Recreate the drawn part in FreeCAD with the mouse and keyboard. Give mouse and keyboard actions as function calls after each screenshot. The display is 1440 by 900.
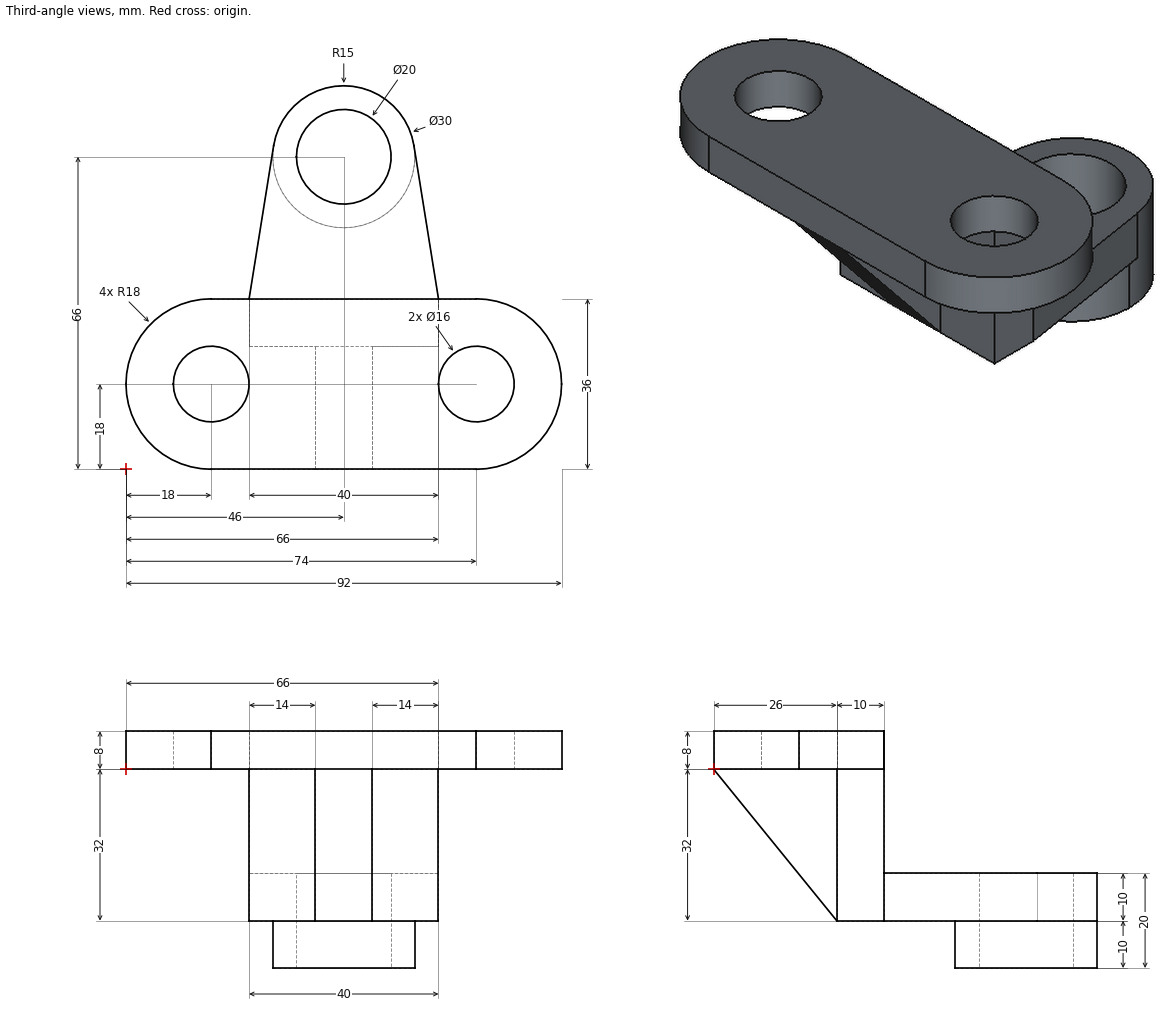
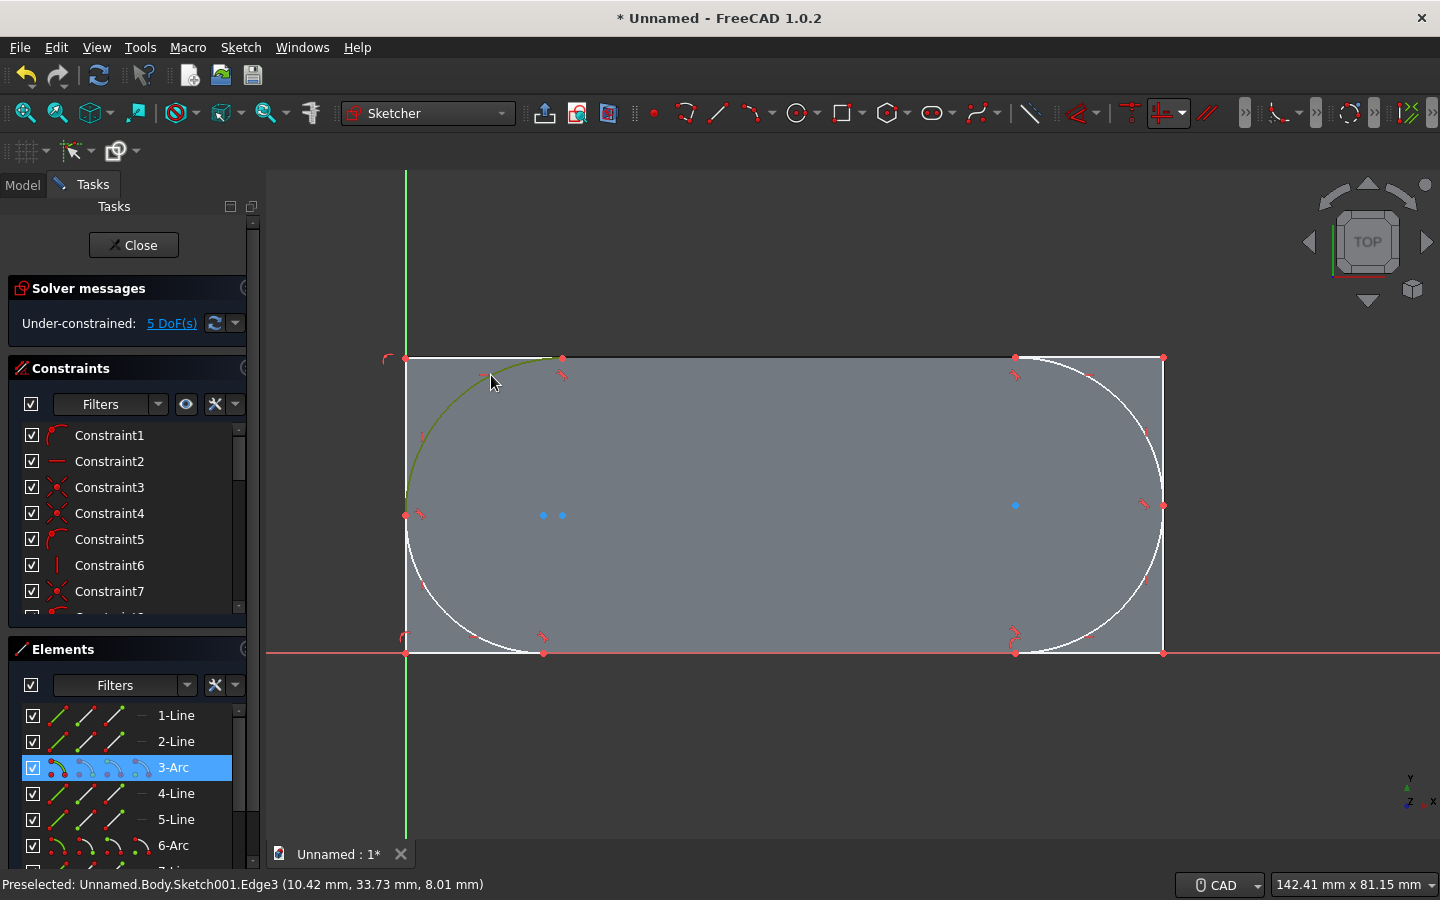
click(481, 638)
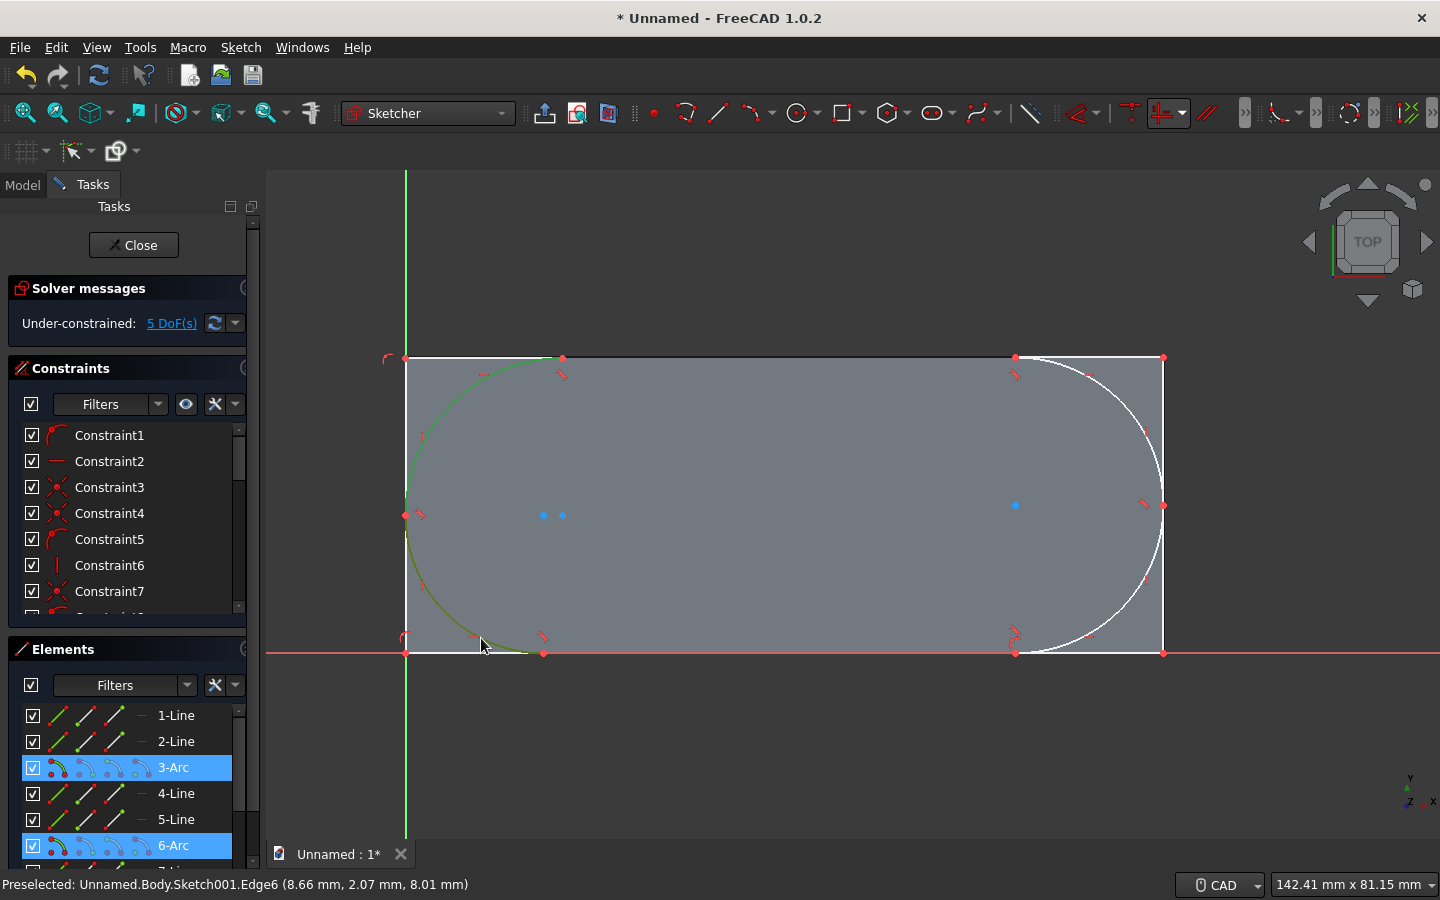
click(1083, 637)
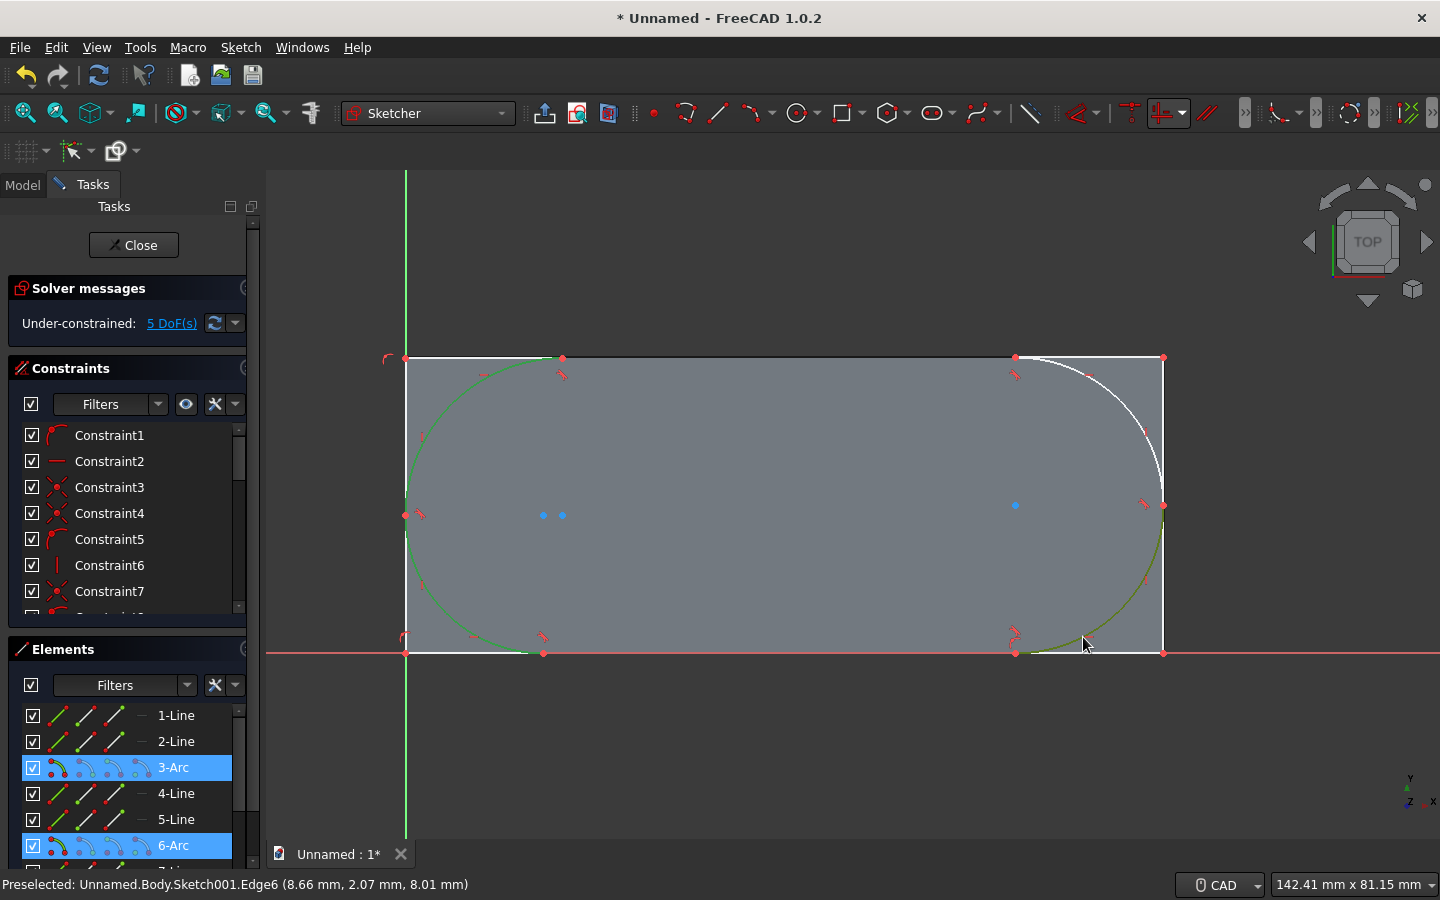
click(1147, 438)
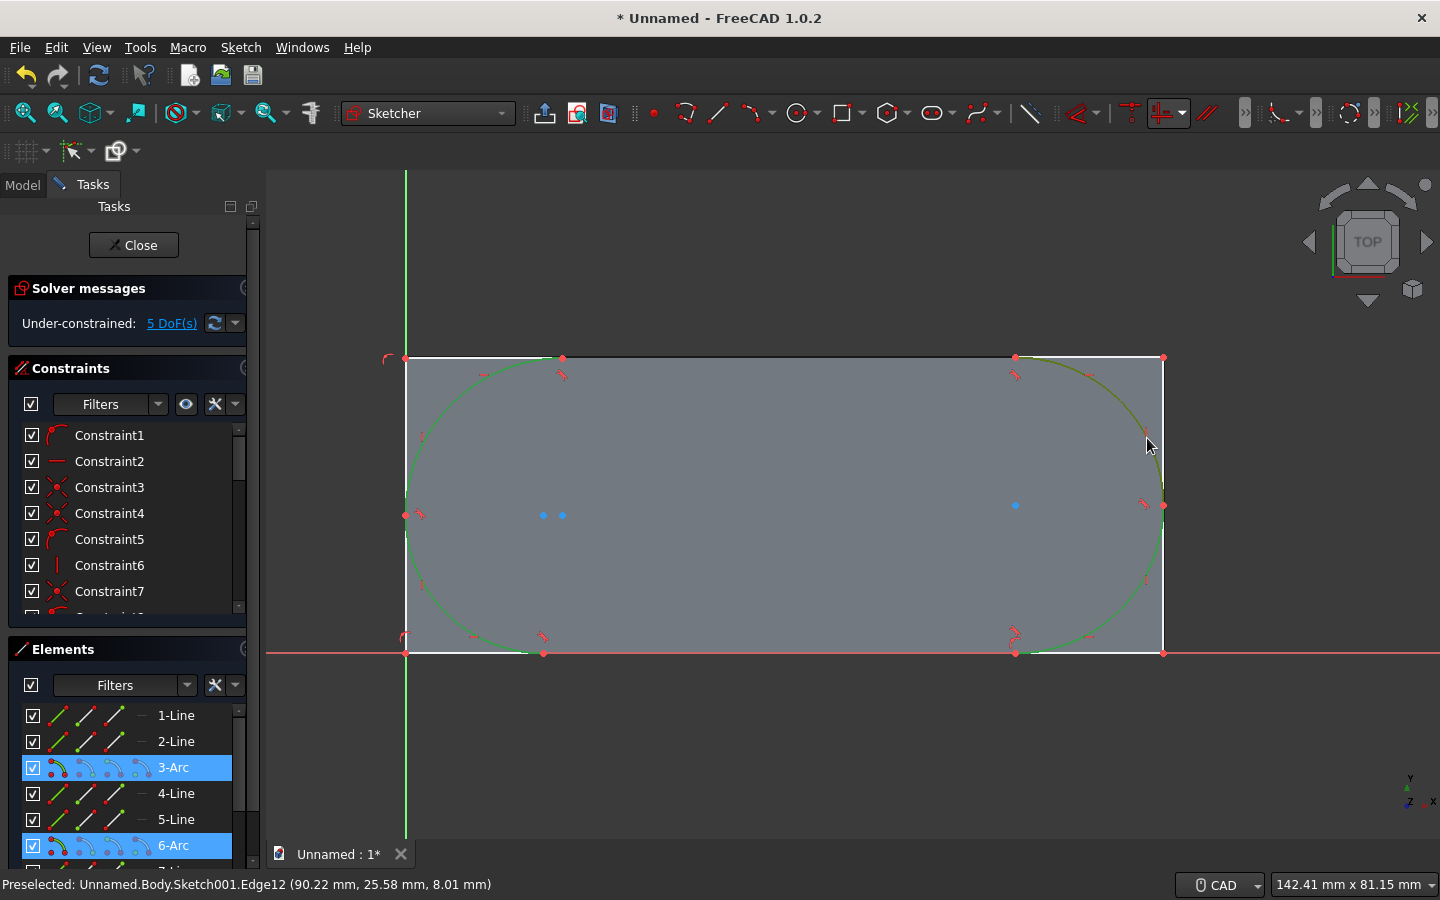
key(e)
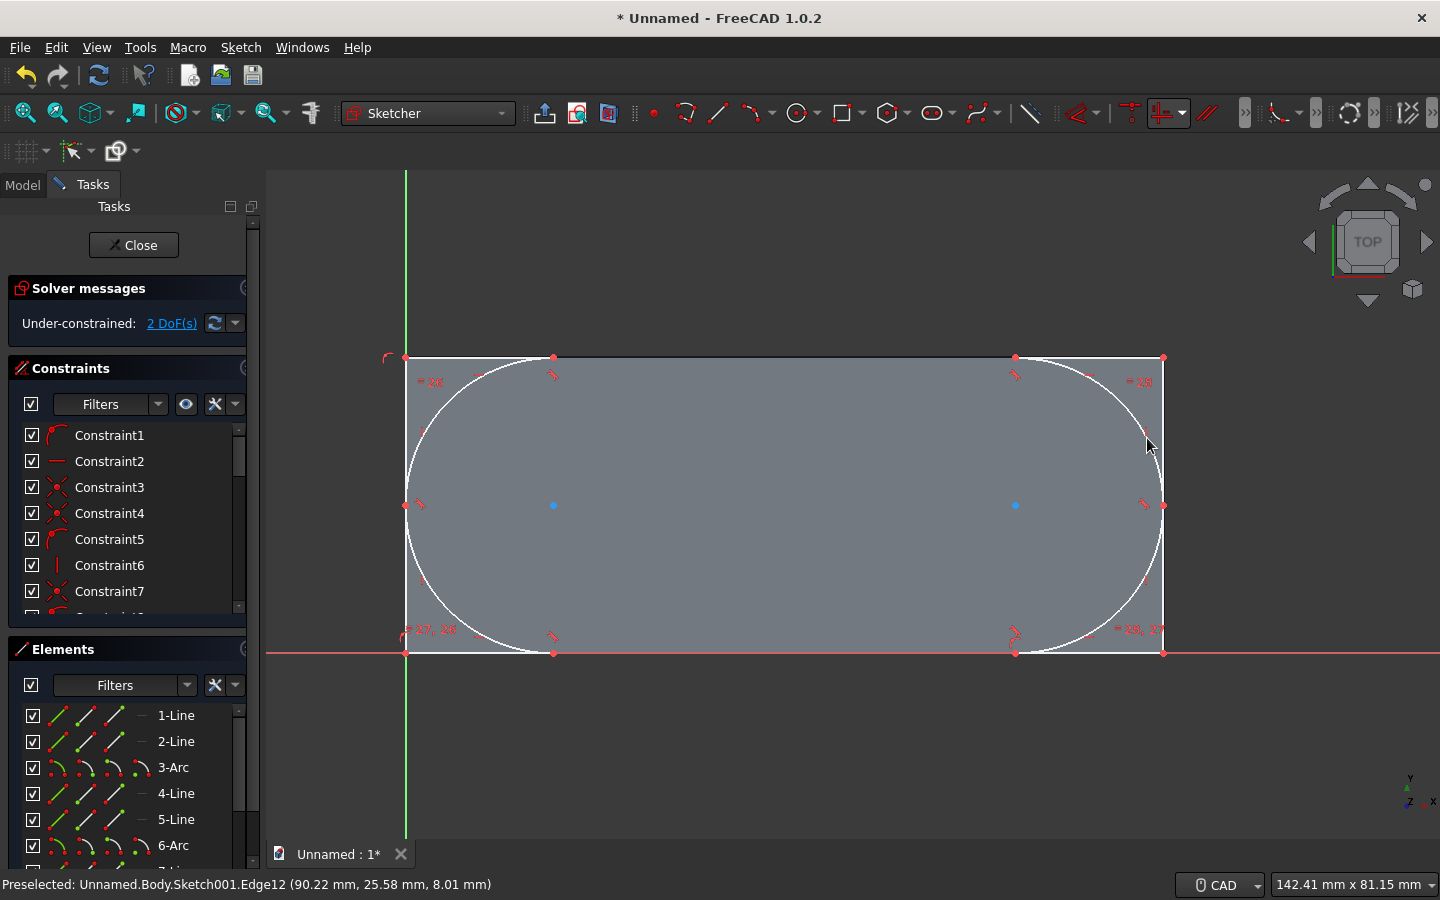
click(1076, 114)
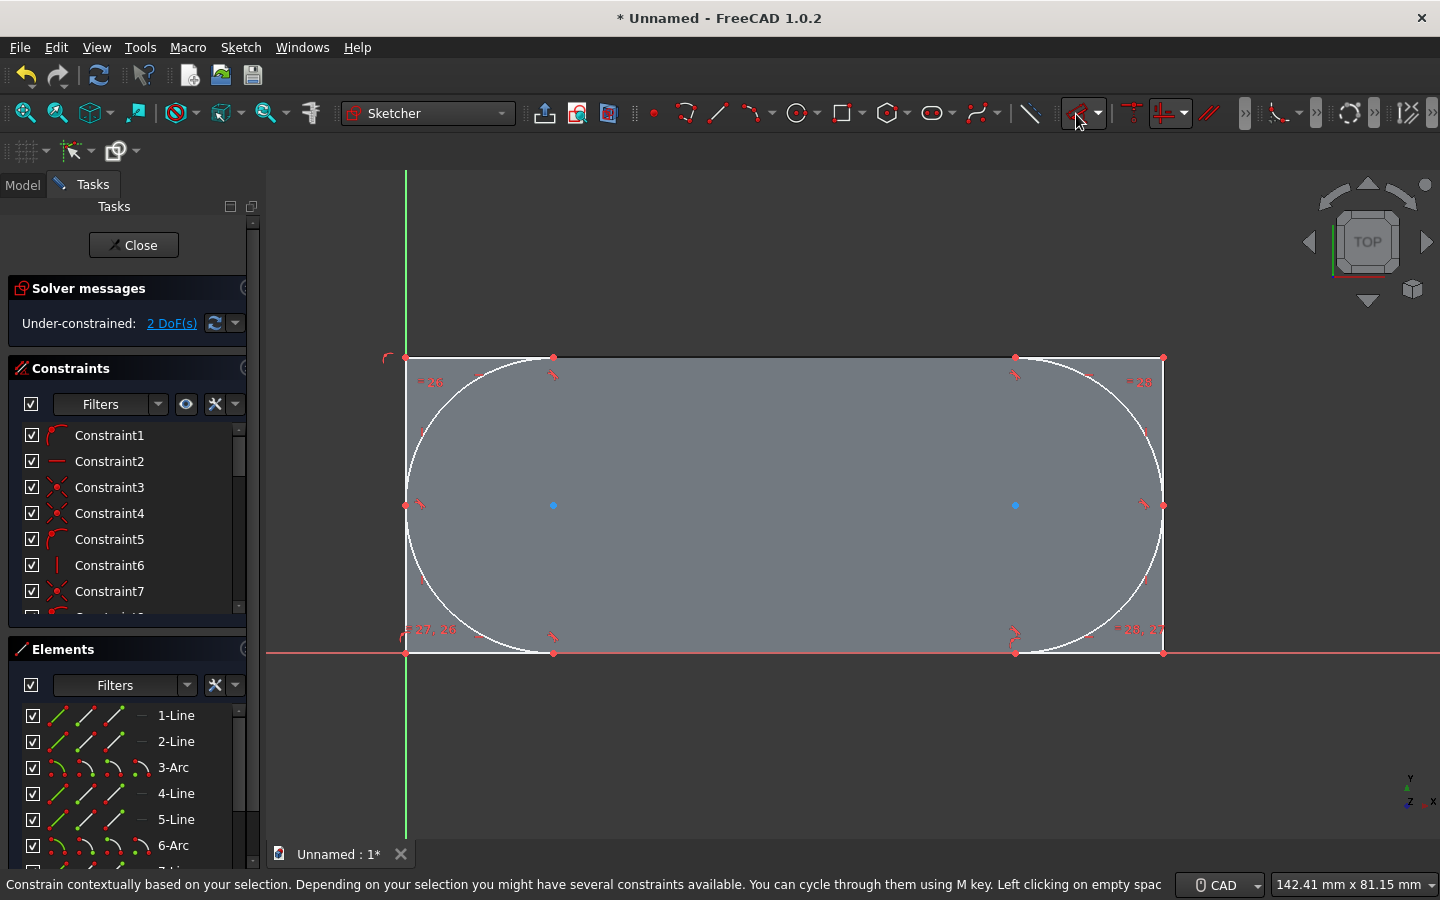
click(486, 374)
click(558, 326)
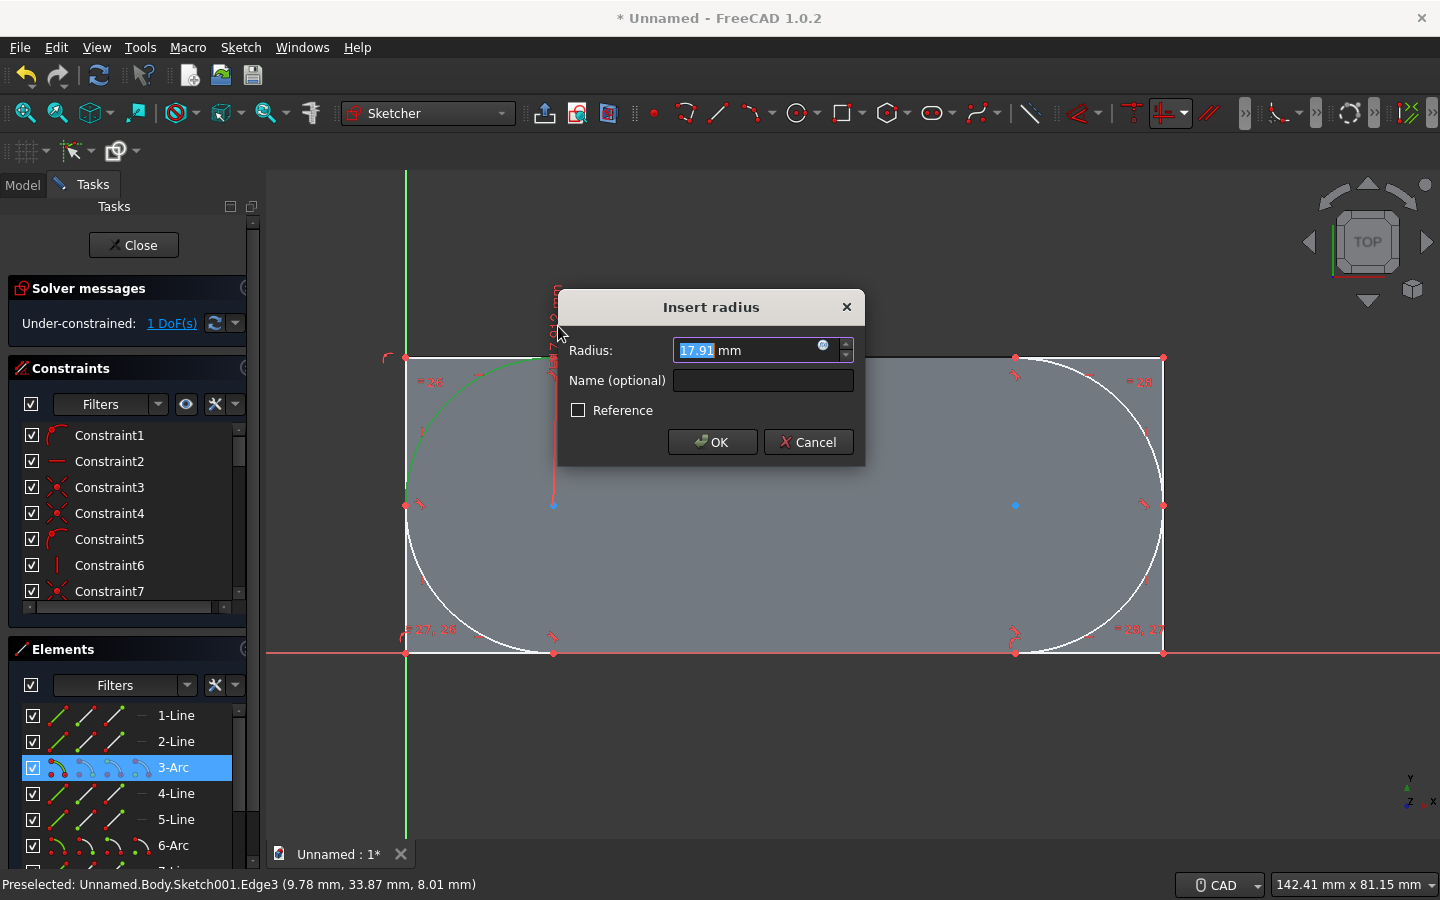
text(18)
key(Return)